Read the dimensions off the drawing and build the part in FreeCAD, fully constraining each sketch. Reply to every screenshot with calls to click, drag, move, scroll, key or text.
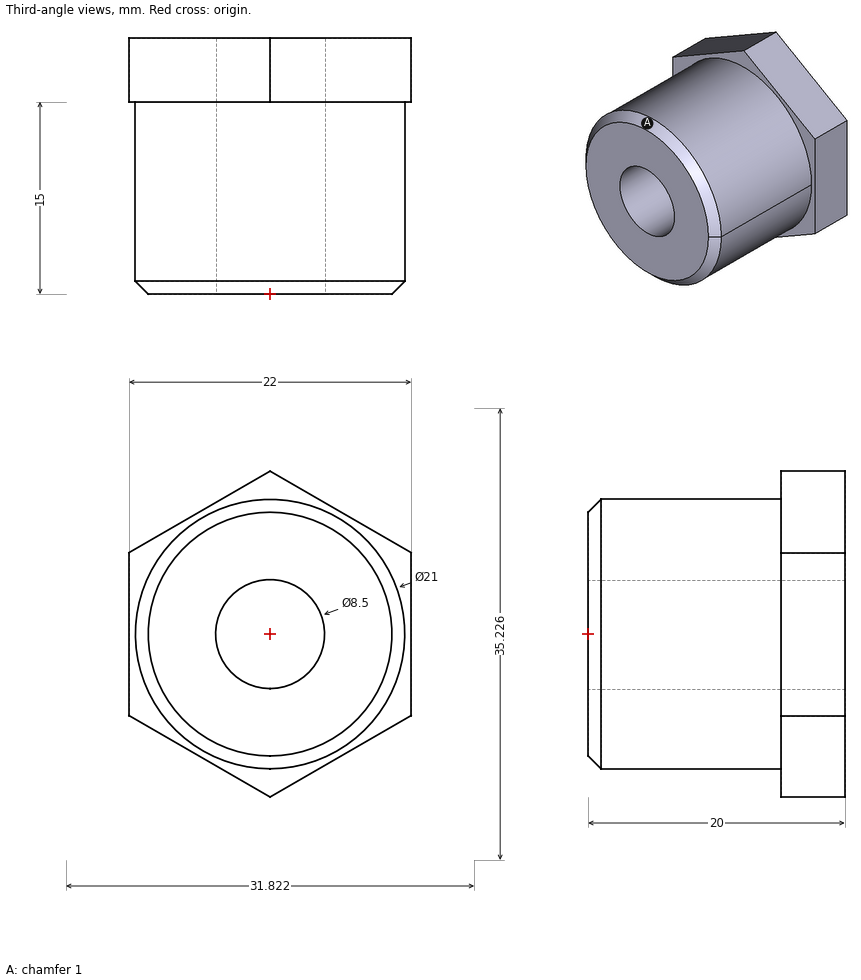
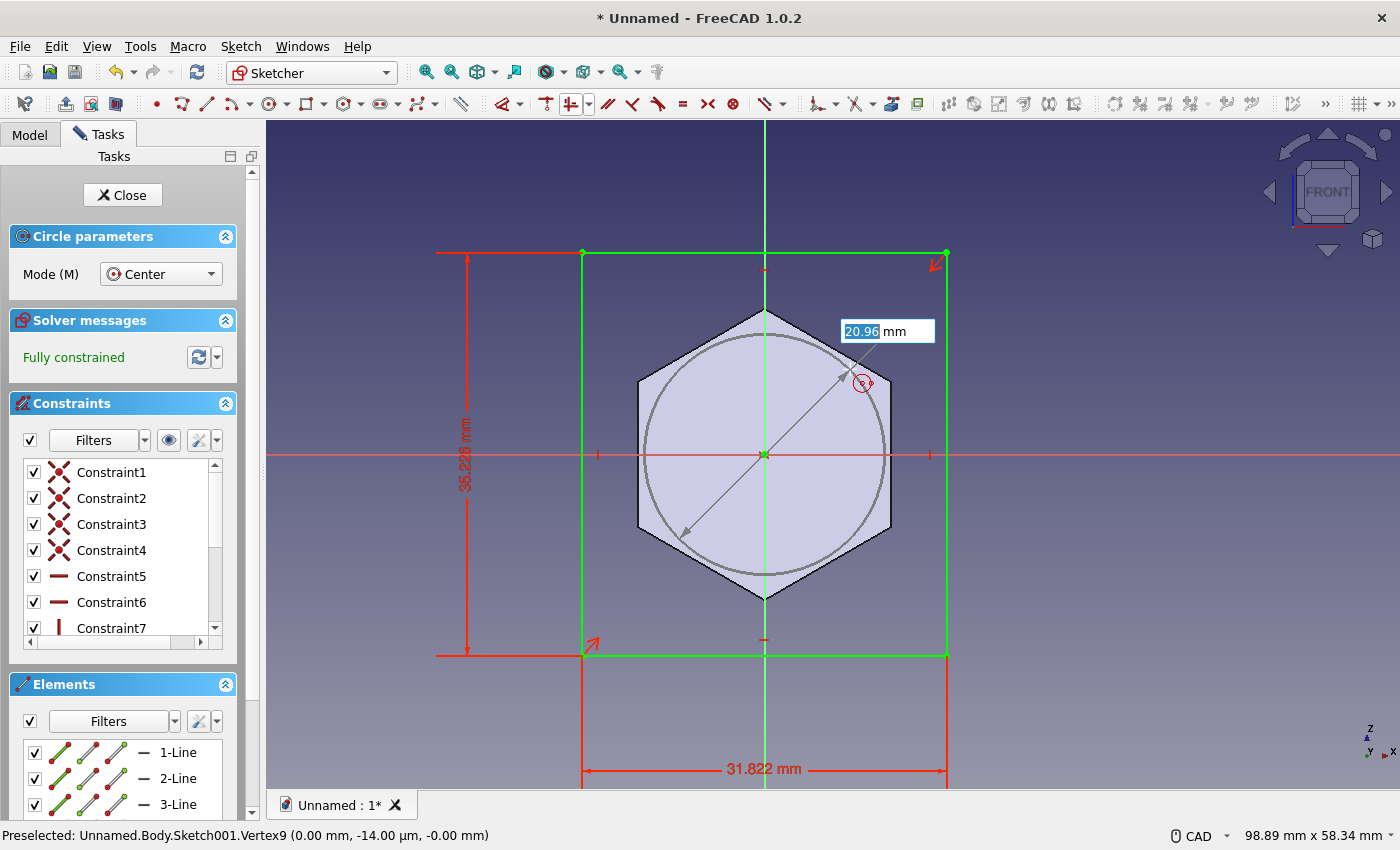
text(21)
key(Return)
key(Escape)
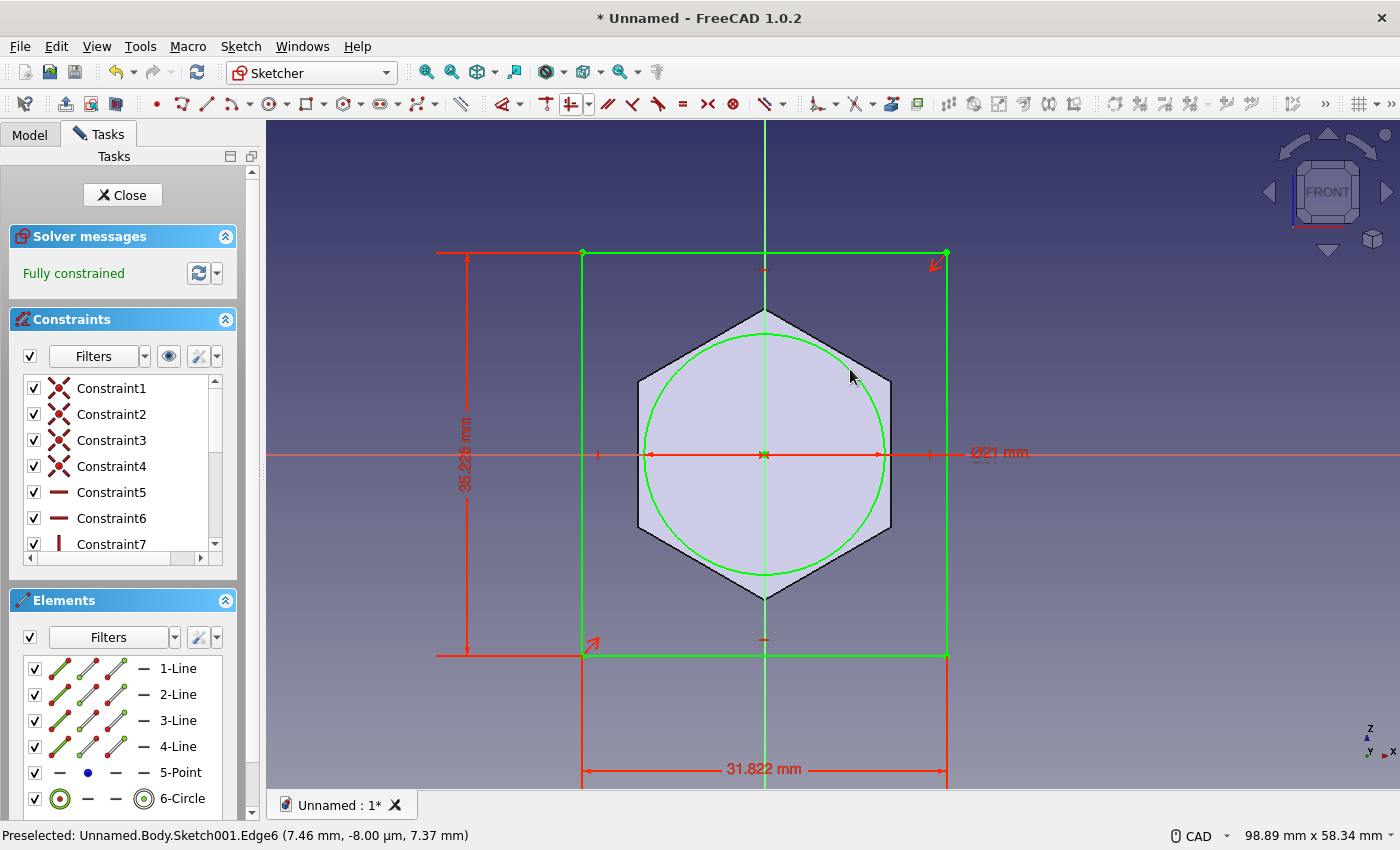
click(123, 195)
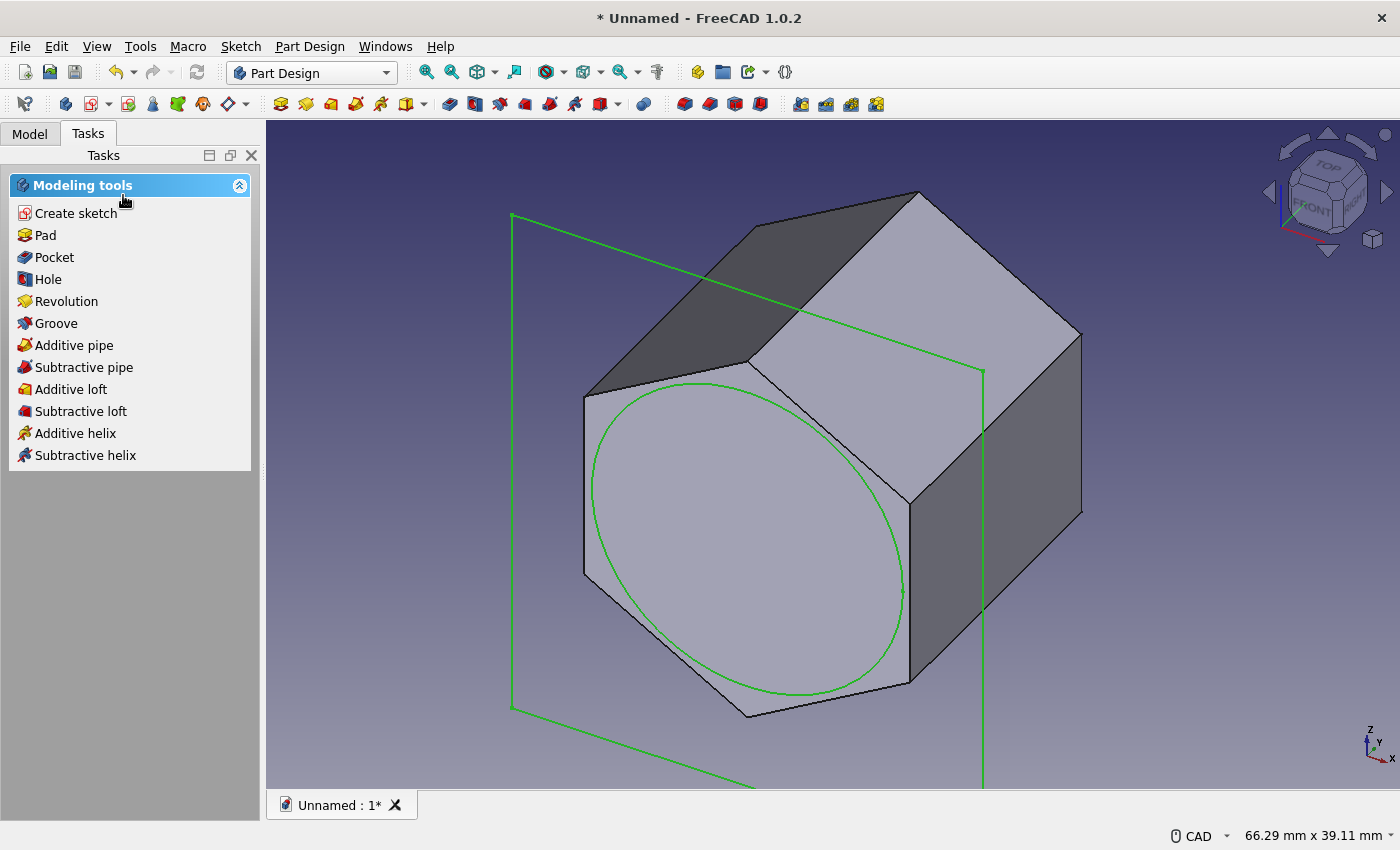
click(450, 104)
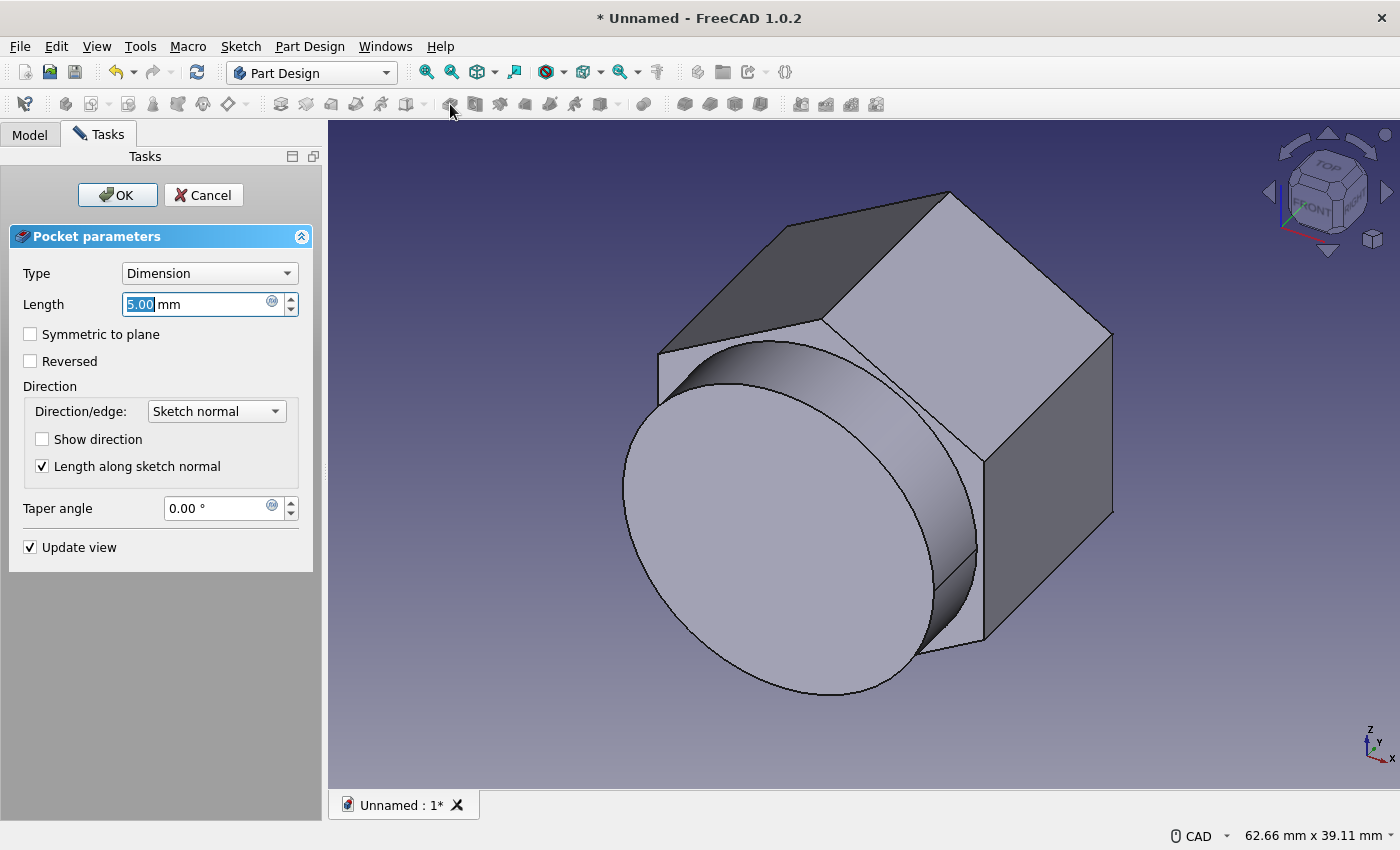
text(15)
key(Tab)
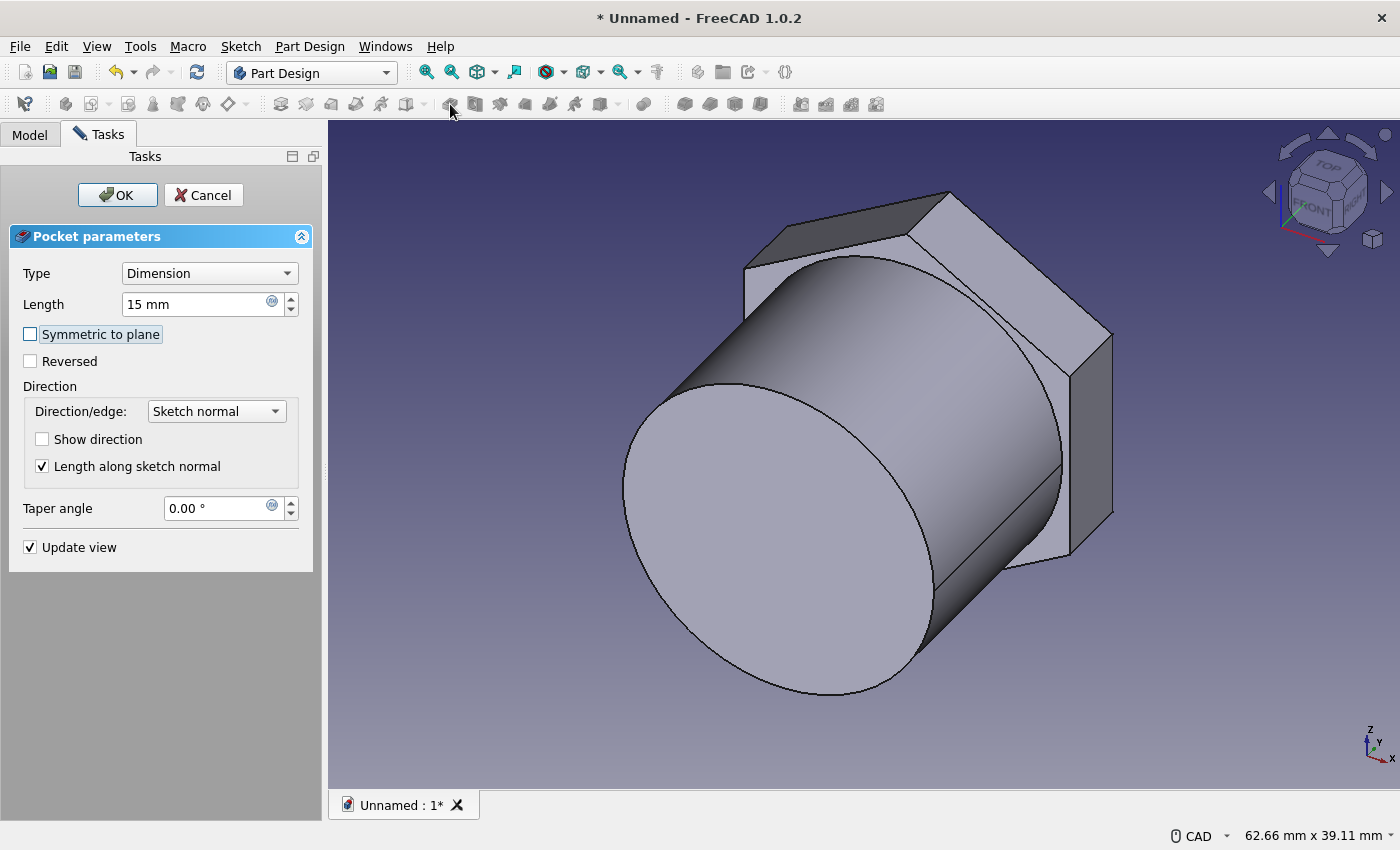
click(118, 195)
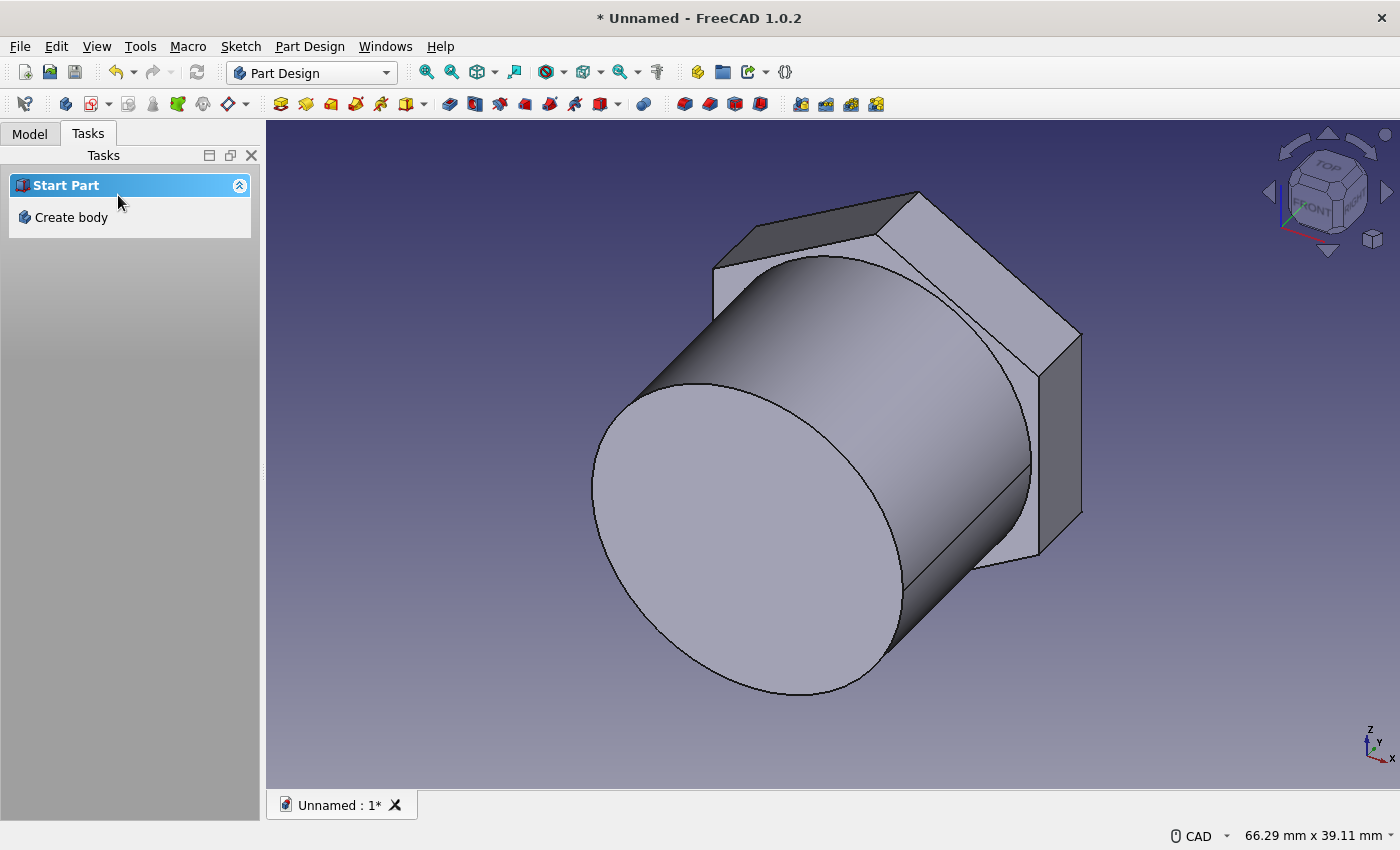
click(622, 410)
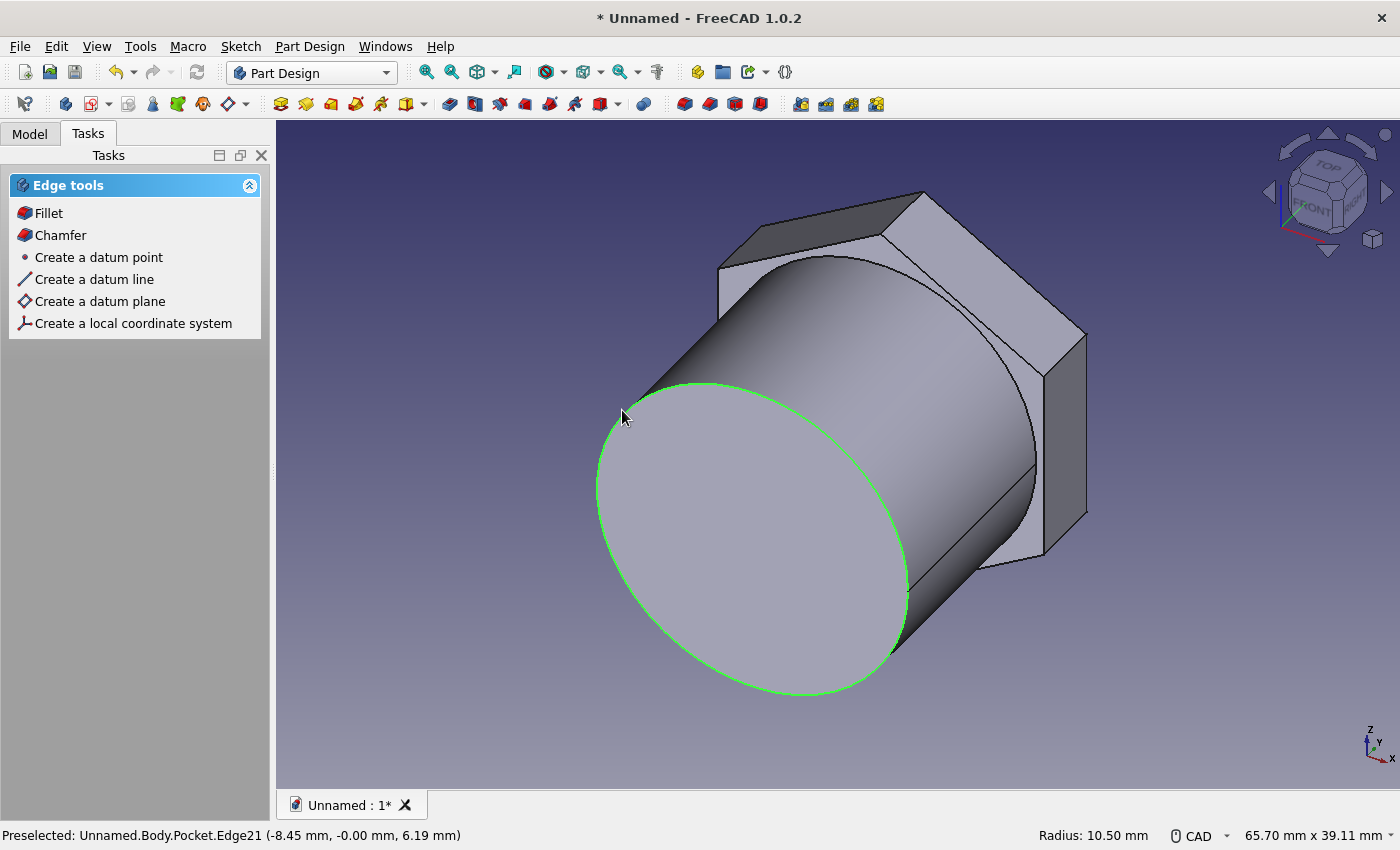
click(710, 104)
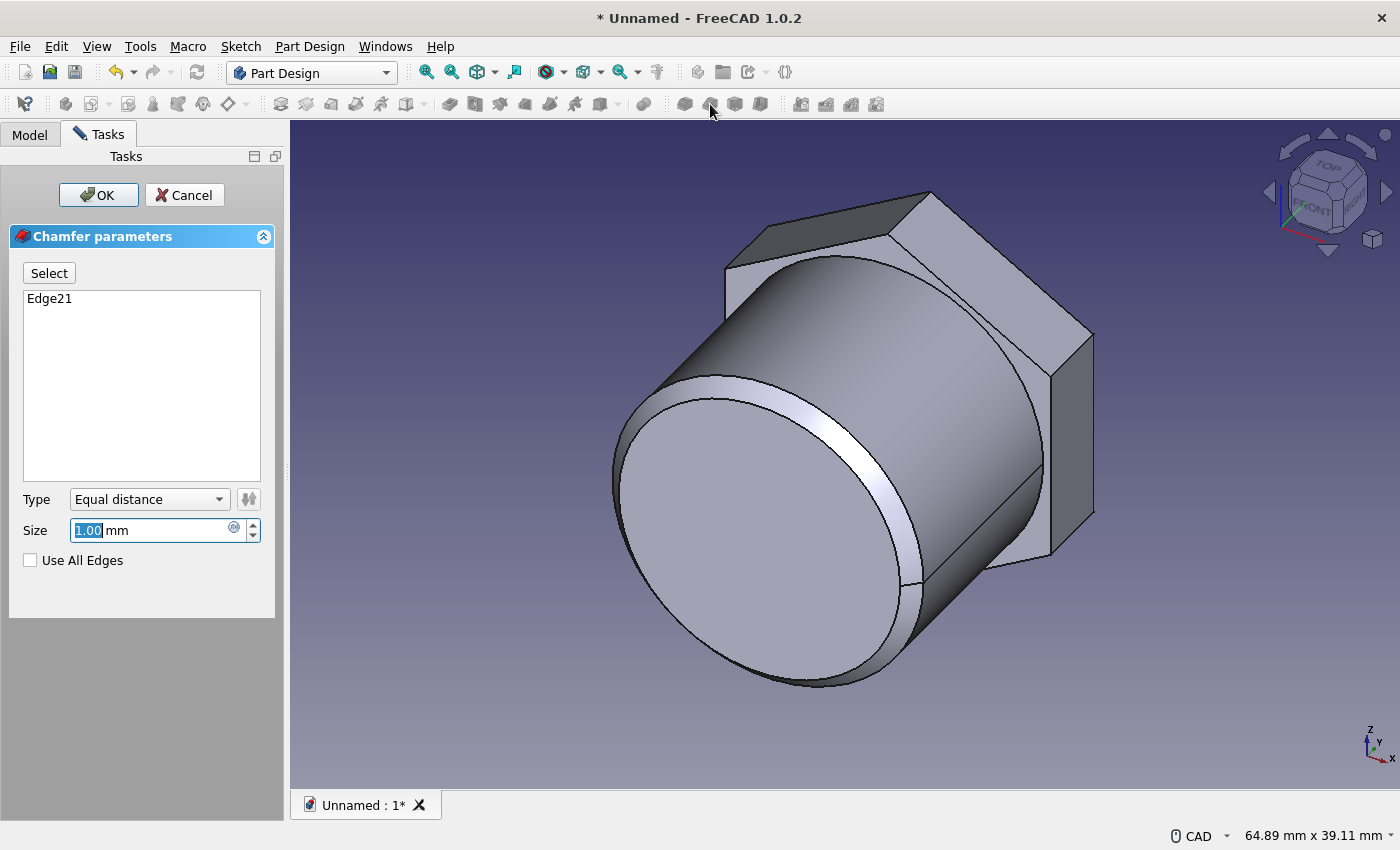
text(1)
key(Tab)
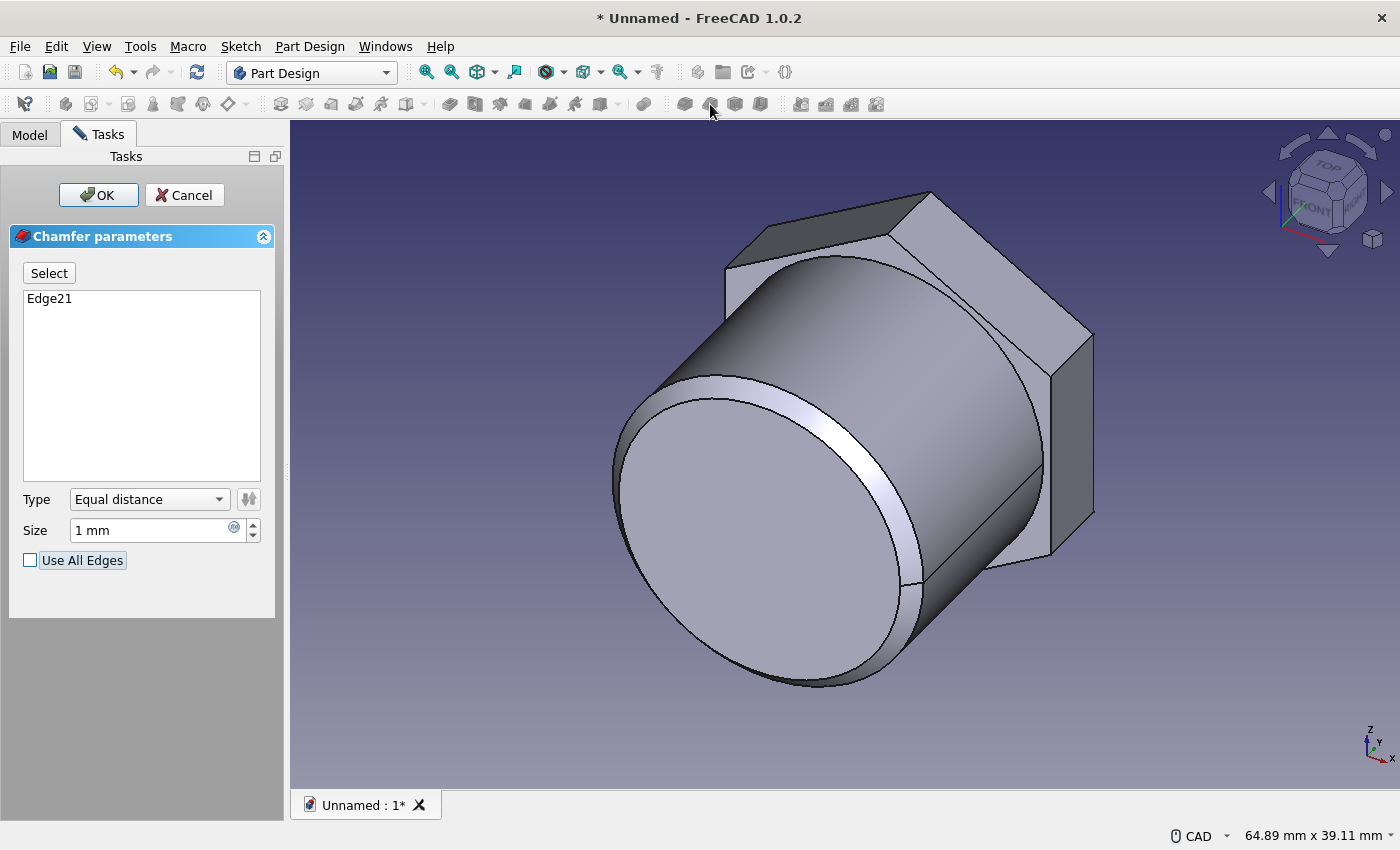
click(99, 195)